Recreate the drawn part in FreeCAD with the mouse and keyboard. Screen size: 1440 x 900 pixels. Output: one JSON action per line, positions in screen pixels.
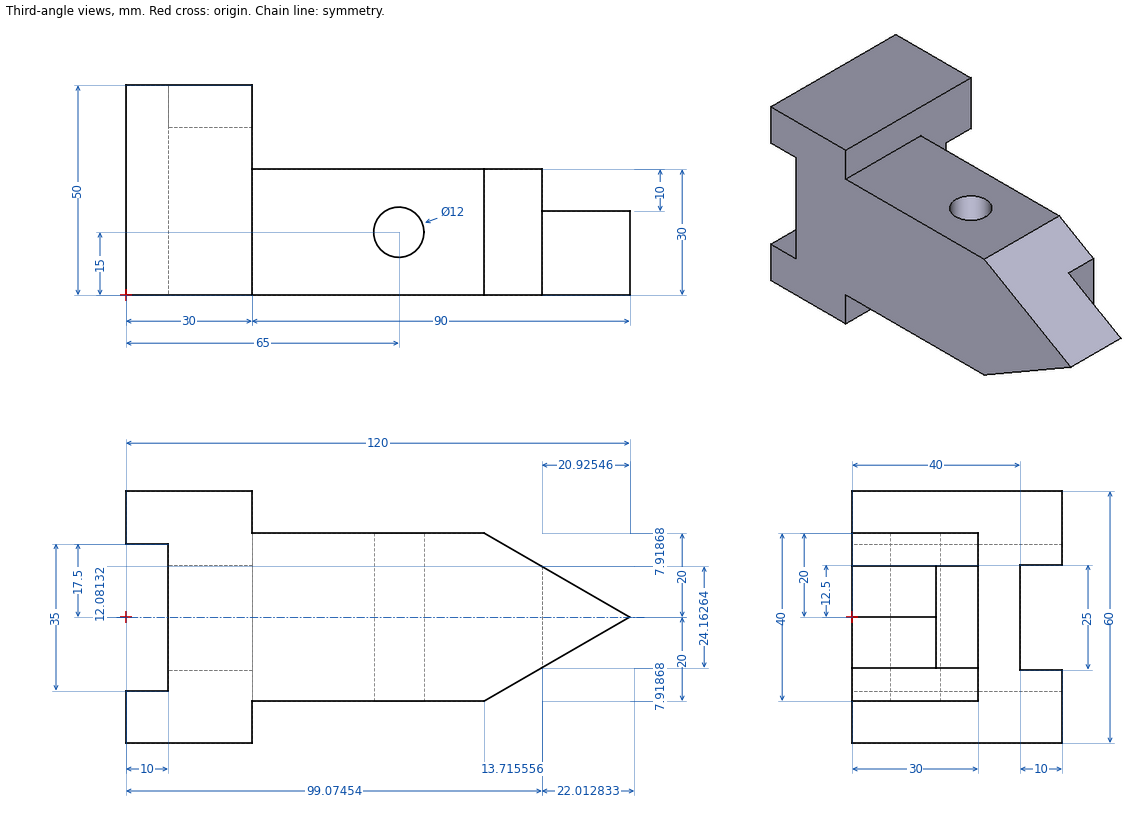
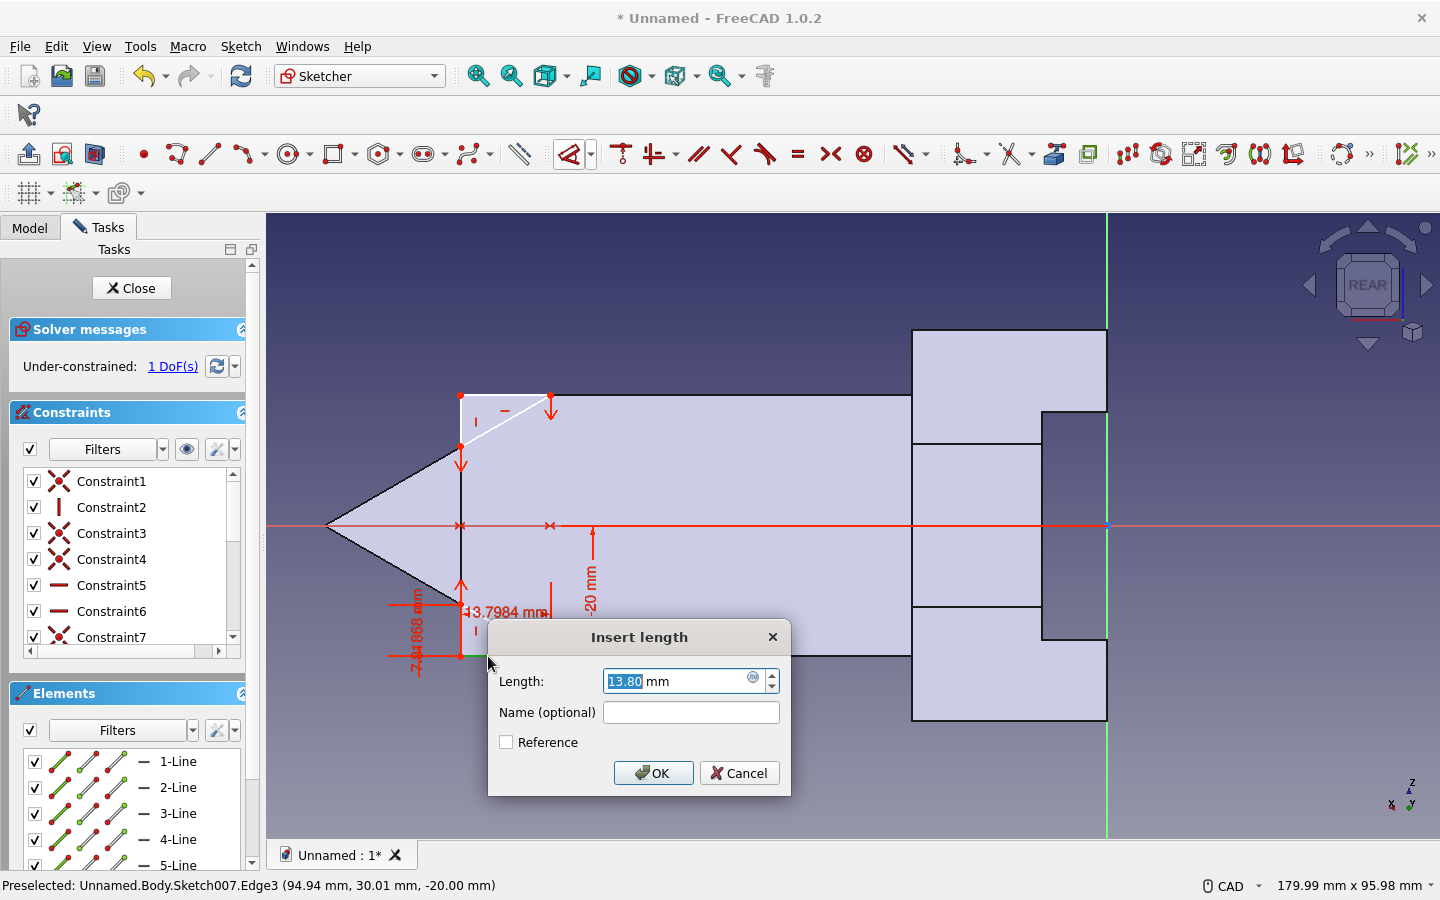
{"action": "type", "text": "13.715556"}
{"action": "key", "text": "Return"}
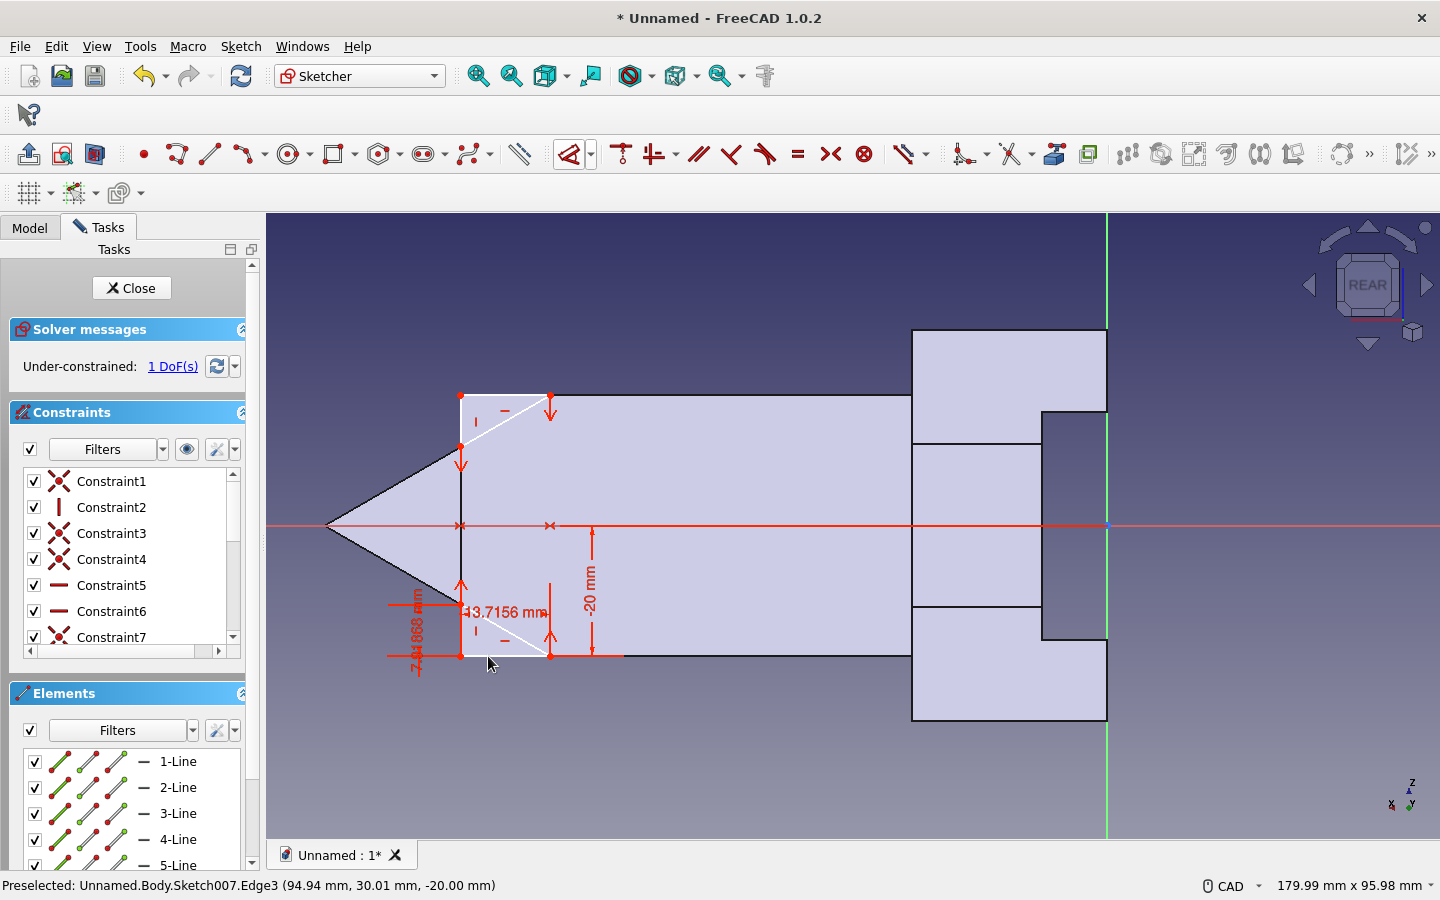
{"action": "left_click", "coordinate": [461, 605]}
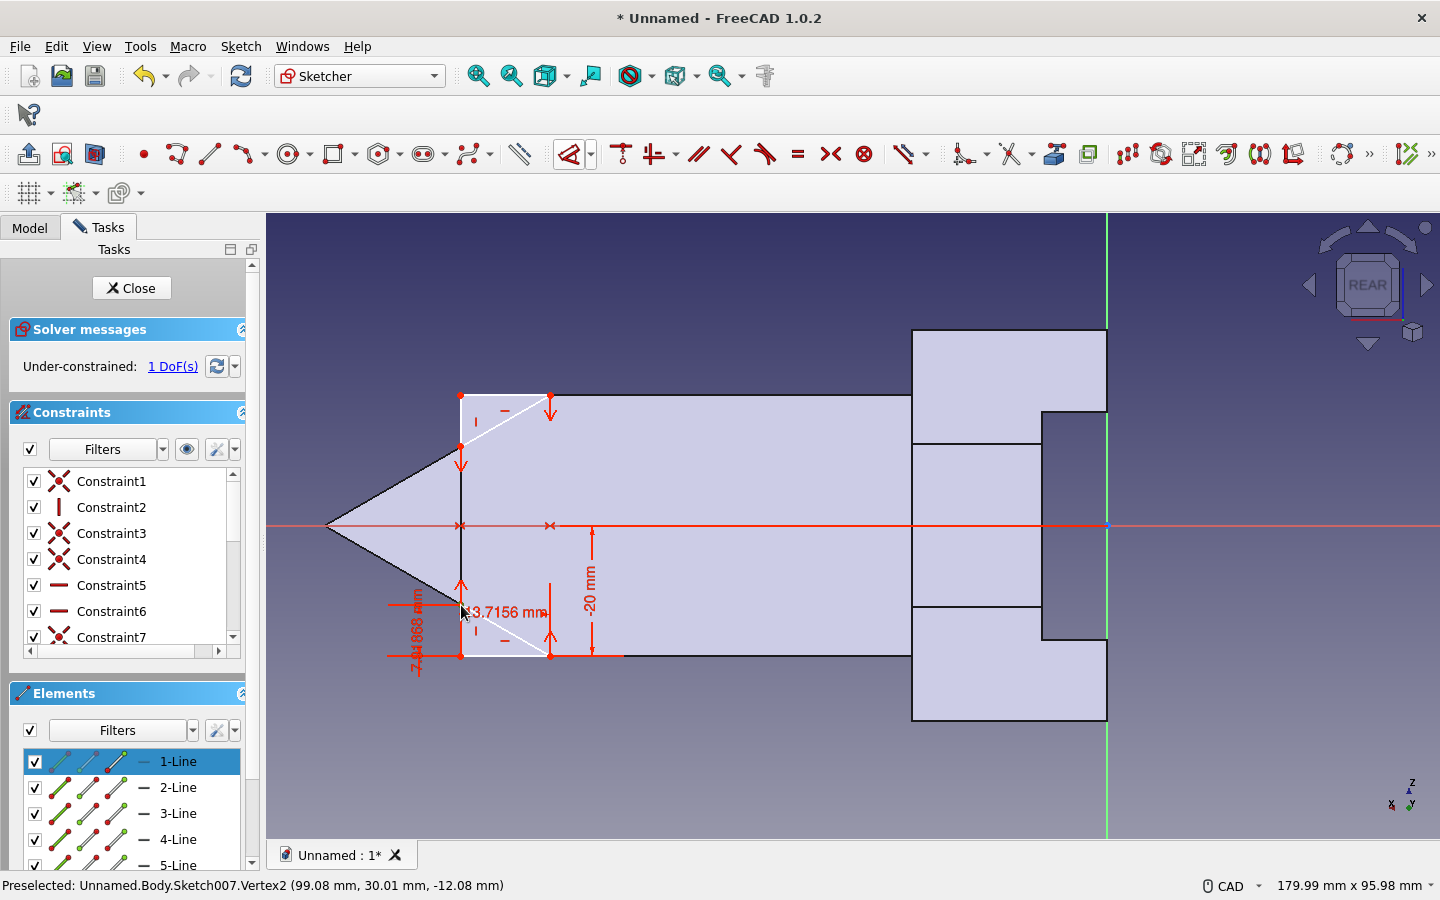
{"action": "left_click", "coordinate": [590, 154]}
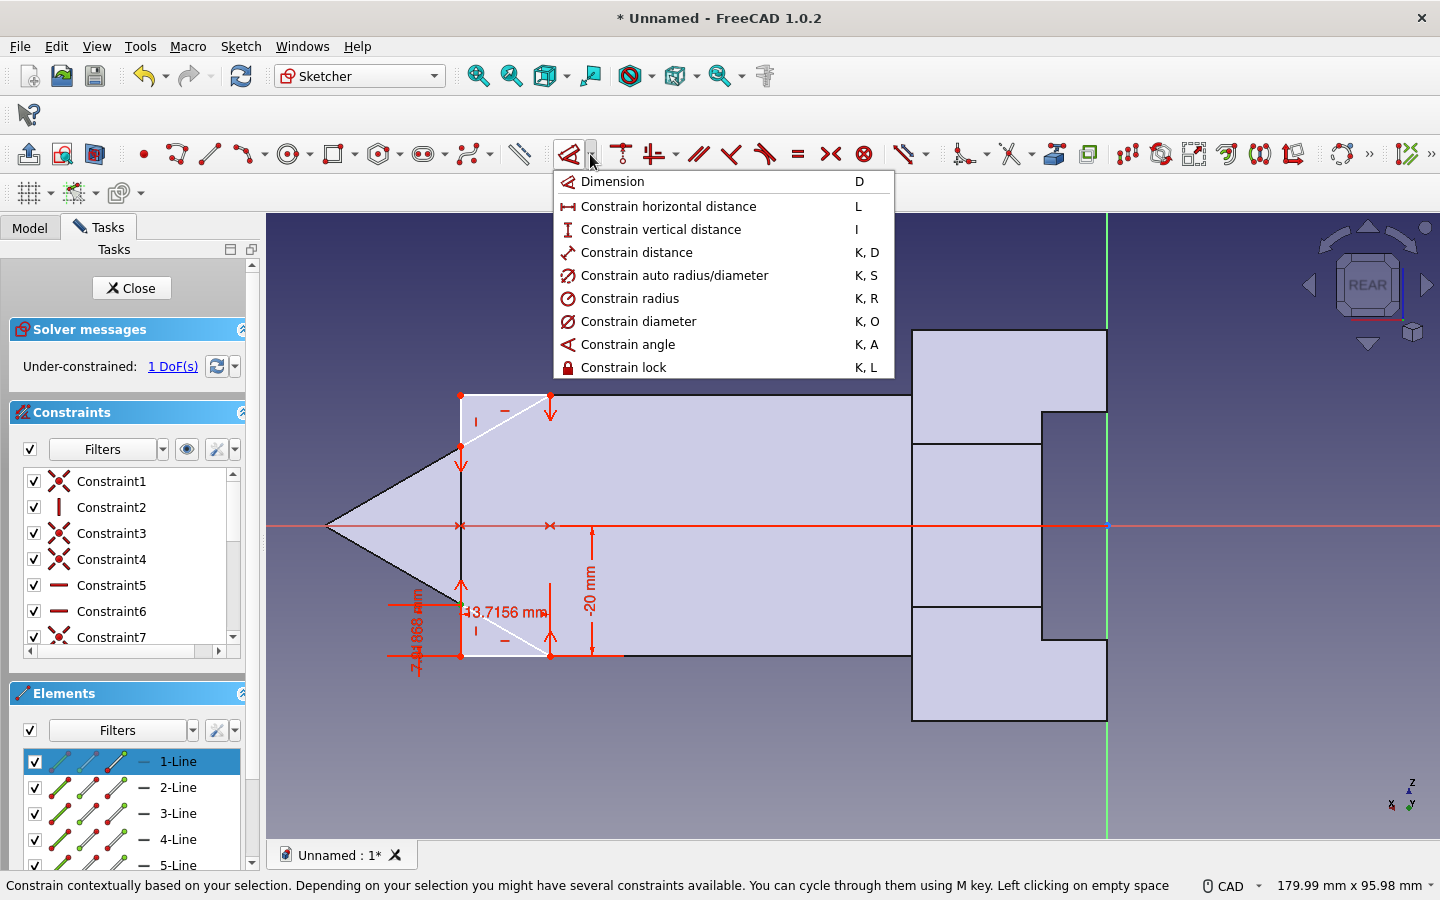
{"action": "left_click", "coordinate": [724, 206]}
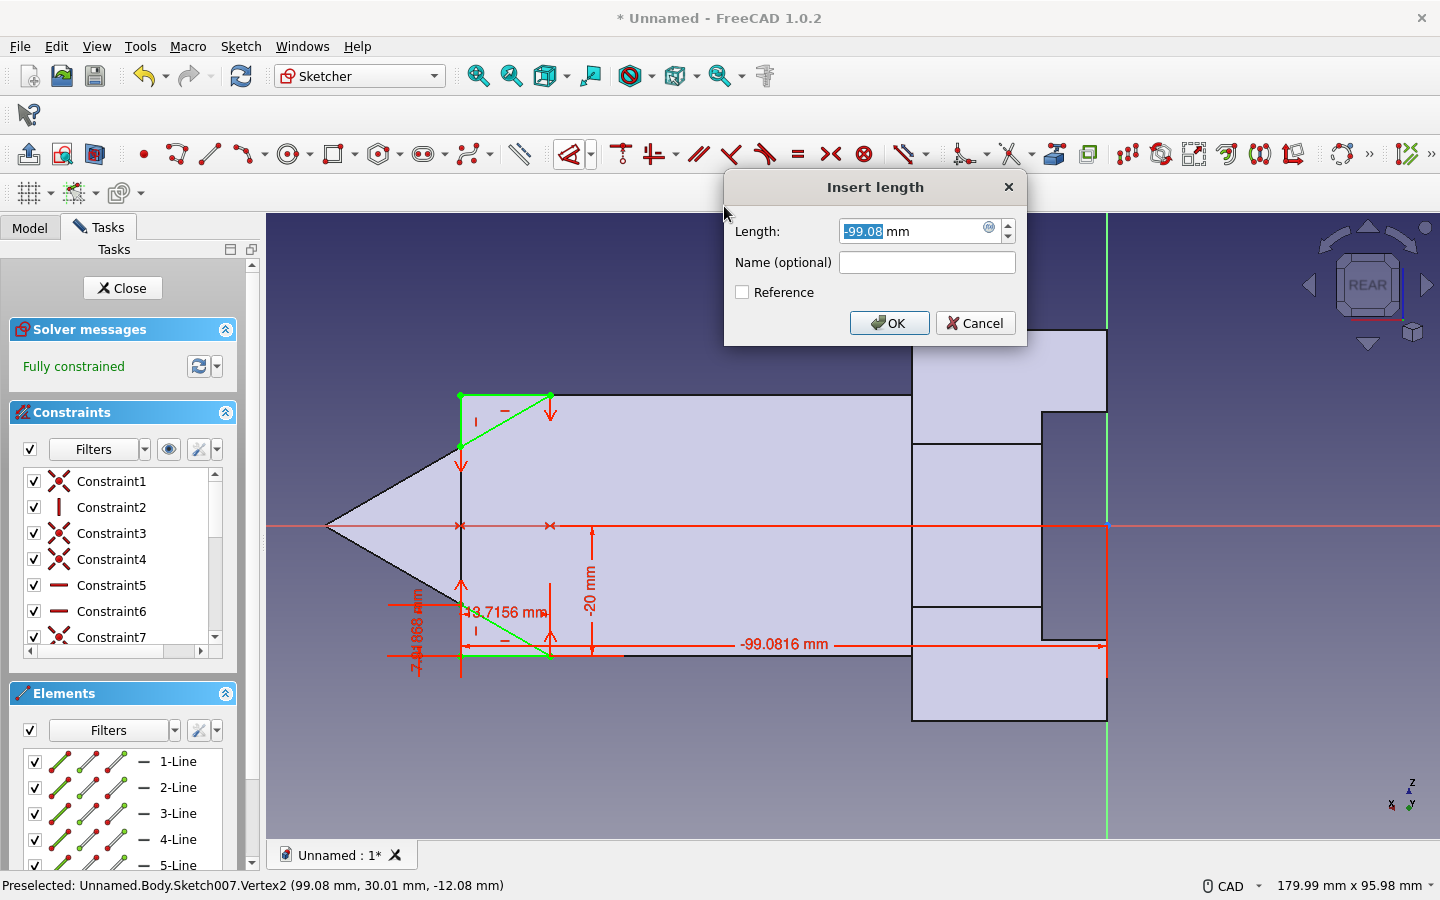
{"action": "type", "text": "-99.07454"}
{"action": "key", "text": "Return"}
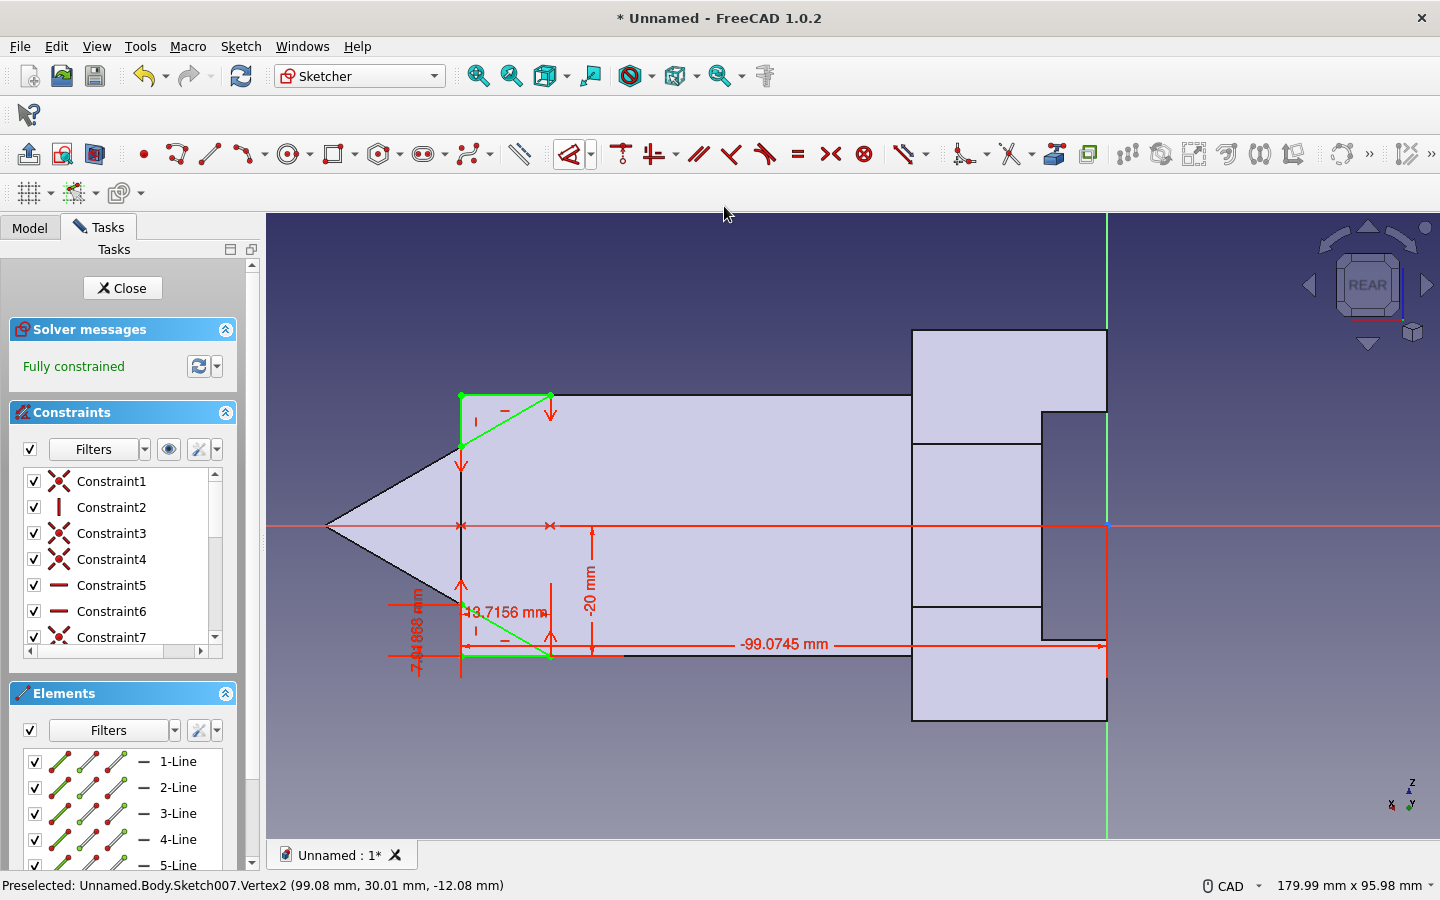
{"action": "left_click", "coordinate": [123, 288]}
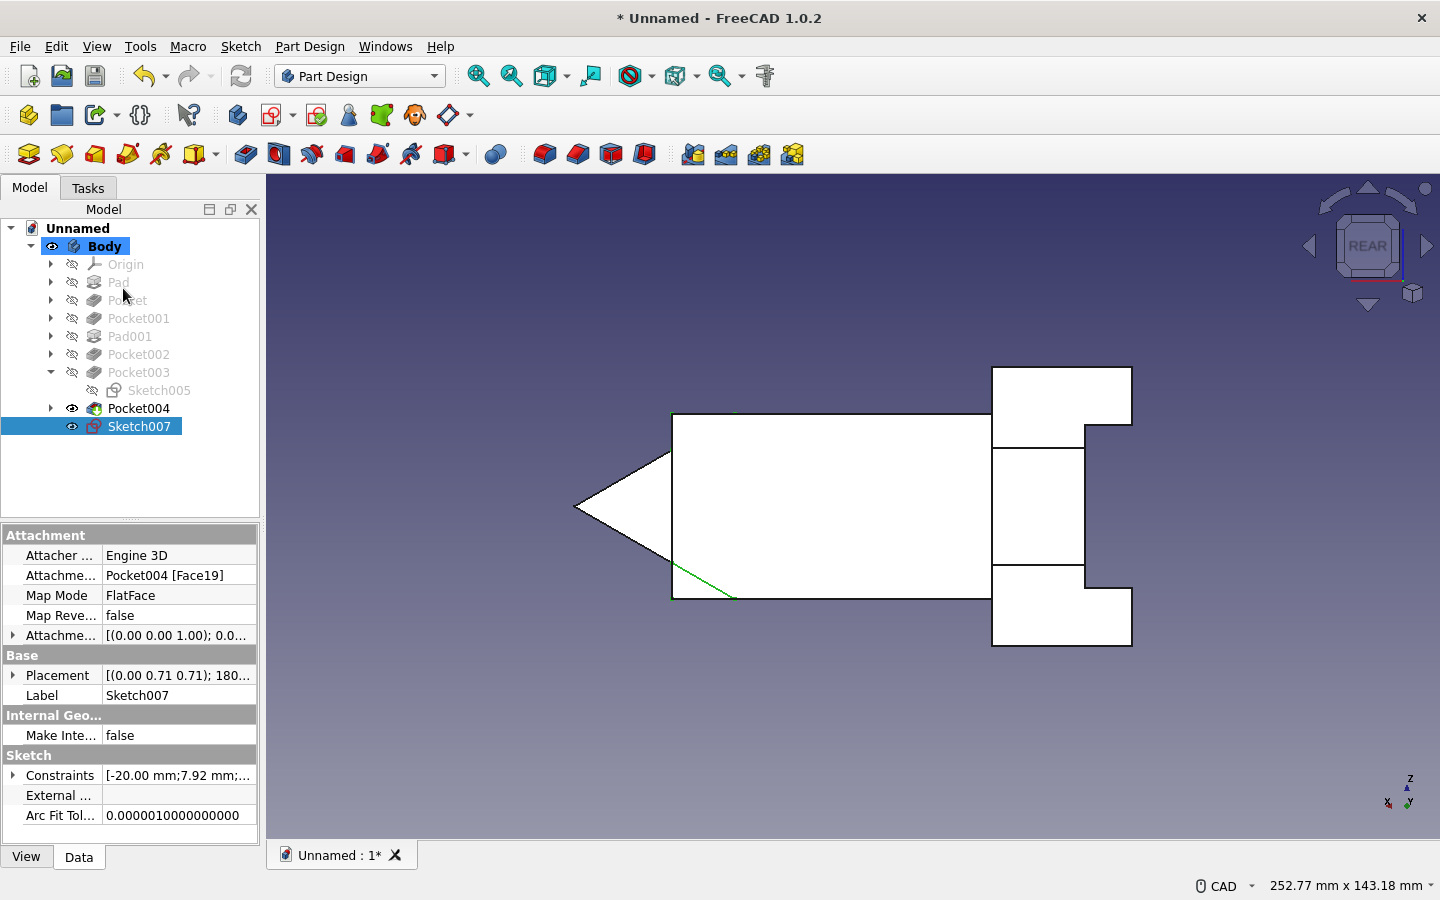
{"action": "left_click", "coordinate": [246, 154]}